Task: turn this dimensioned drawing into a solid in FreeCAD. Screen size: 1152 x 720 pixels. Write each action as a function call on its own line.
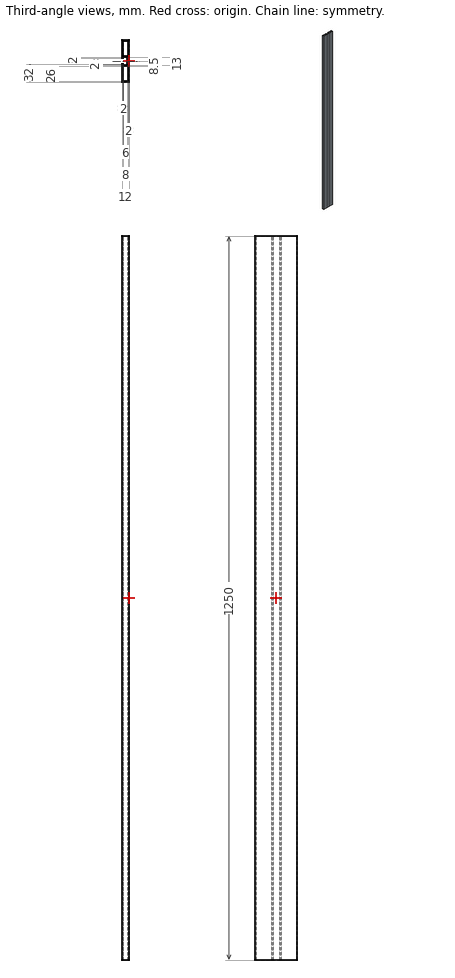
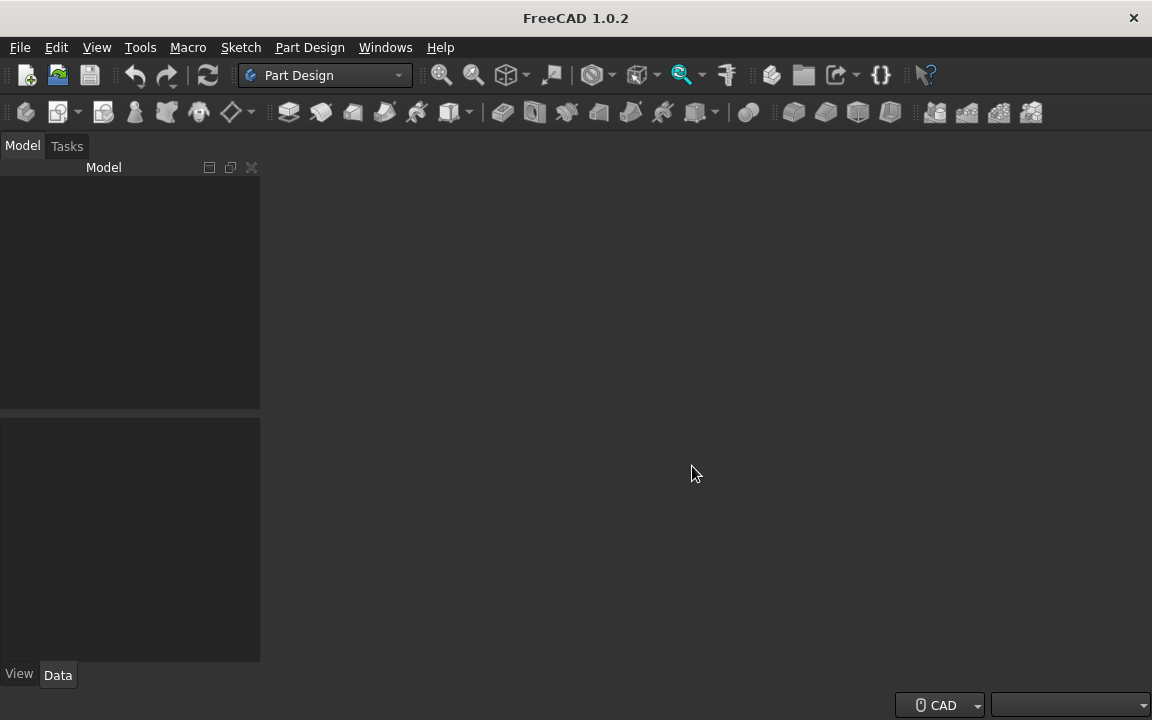
click(26, 76)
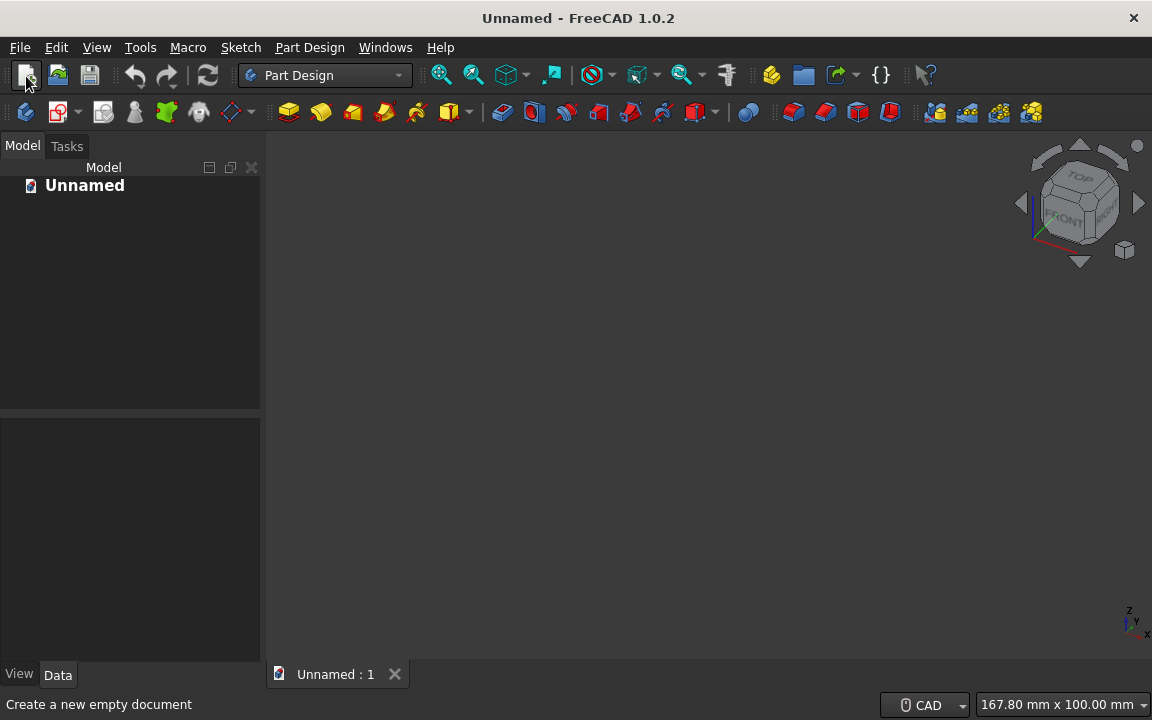
click(58, 112)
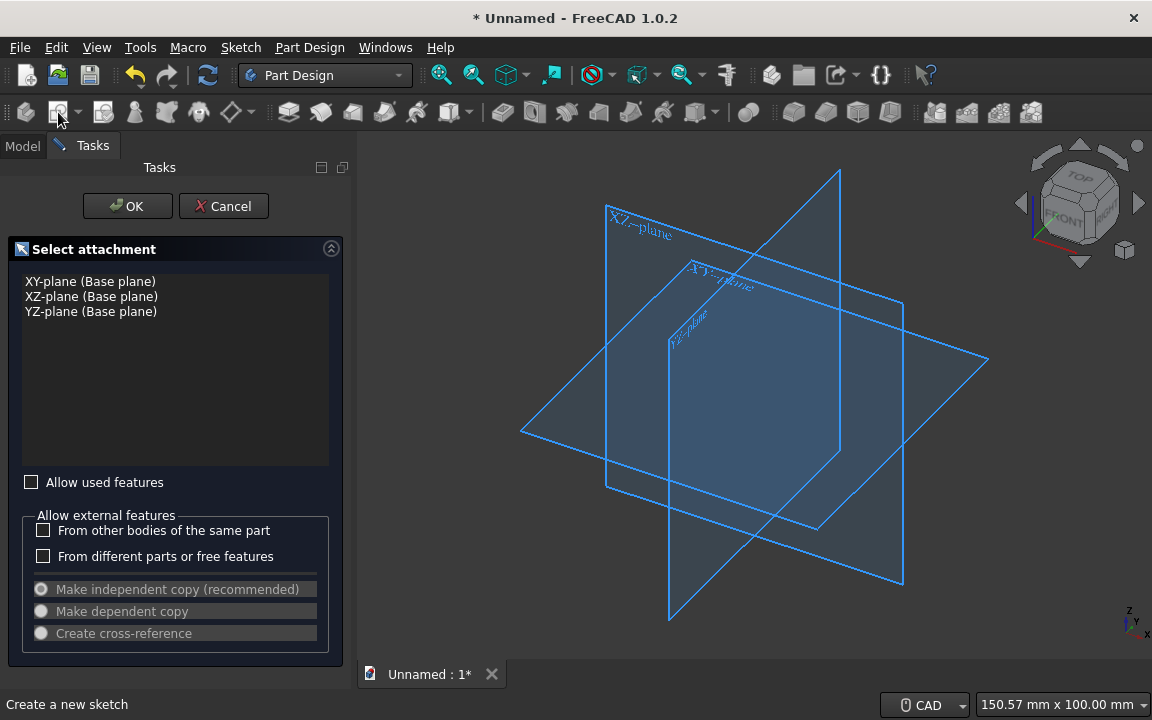
click(82, 282)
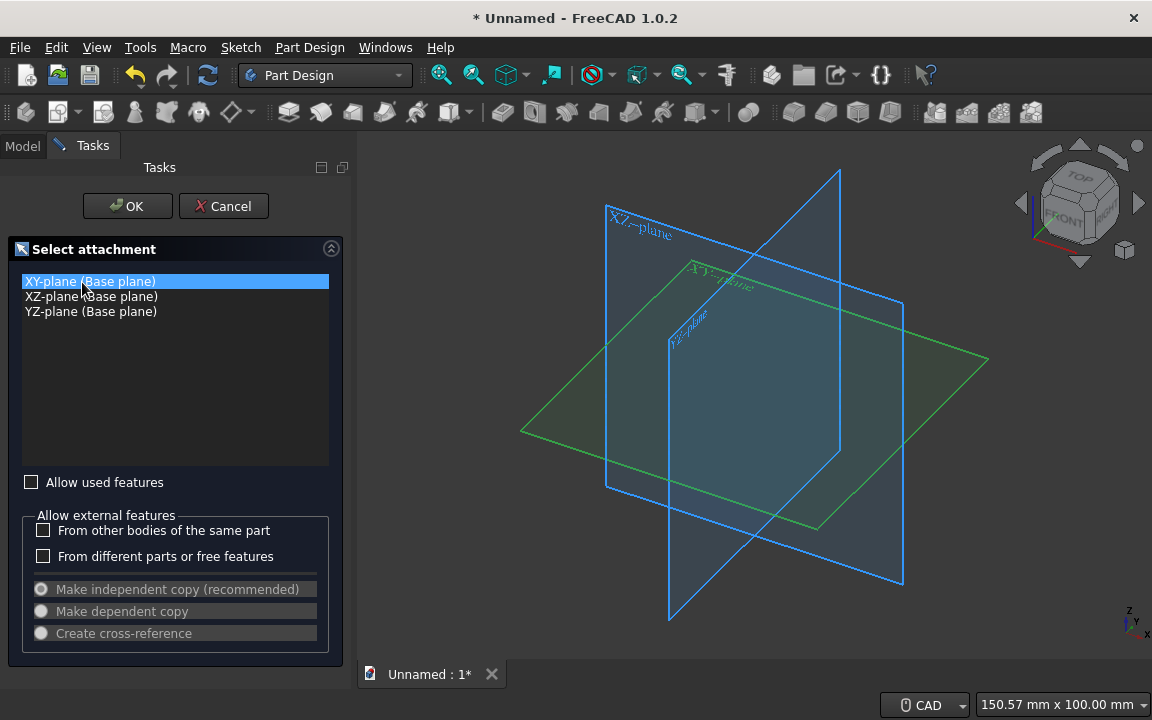
click(128, 206)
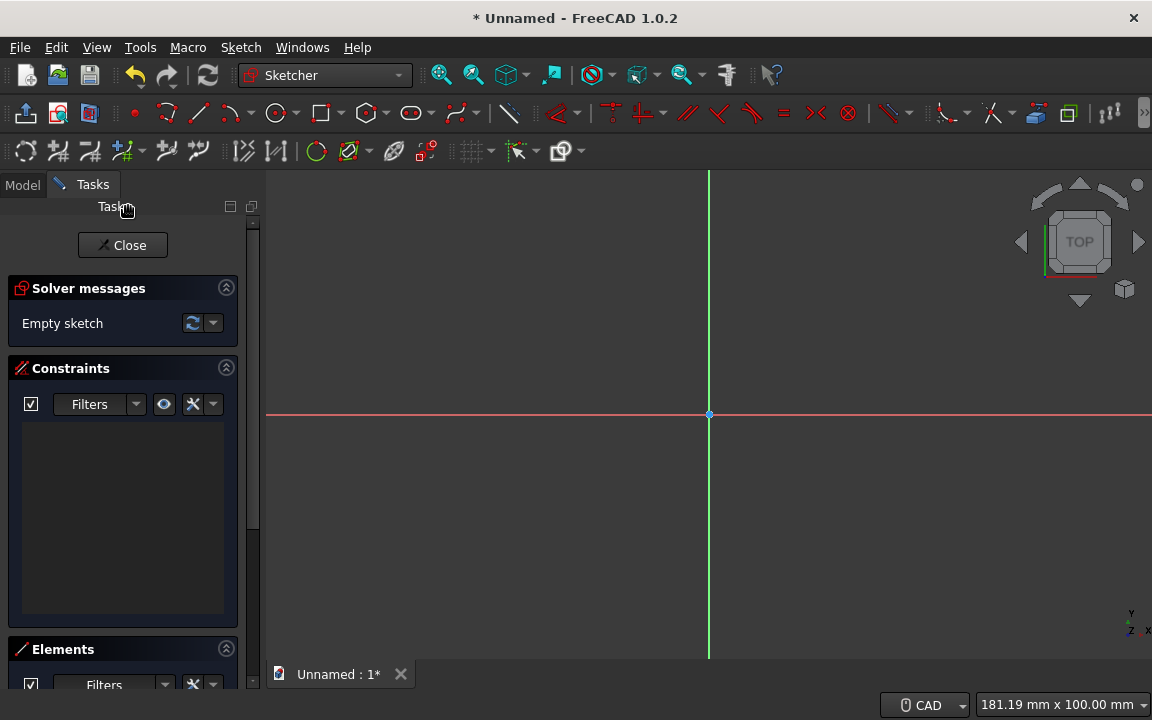
click(168, 114)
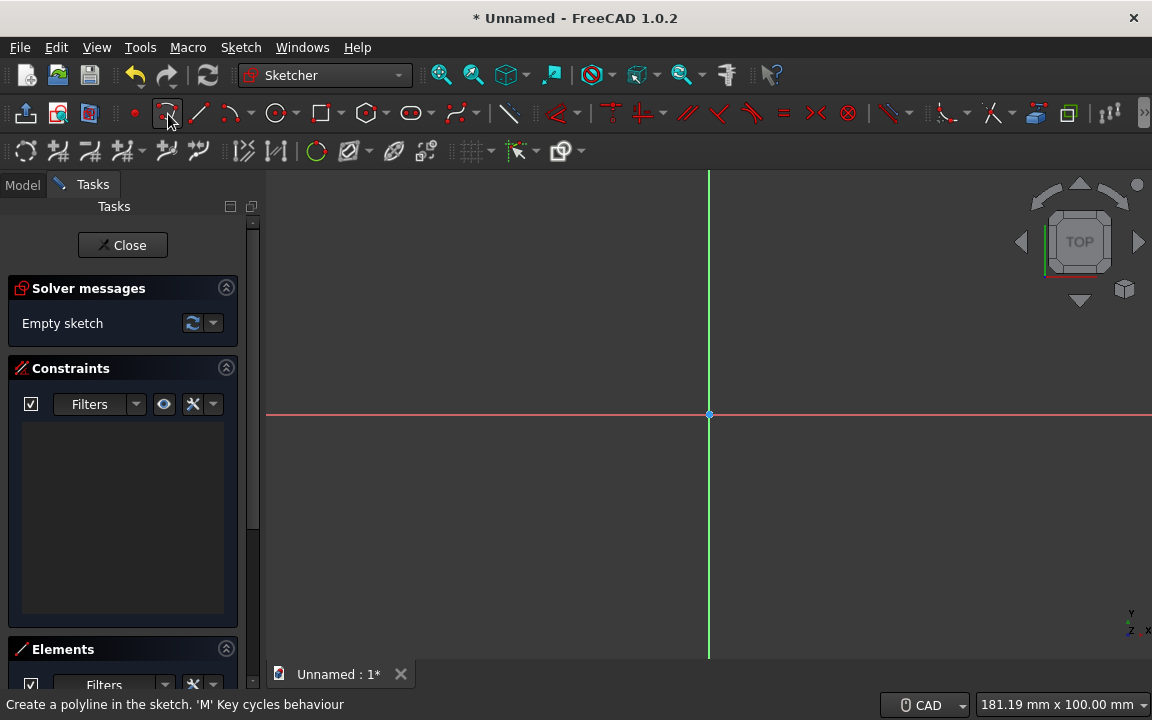
click(689, 383)
click(689, 446)
click(660, 446)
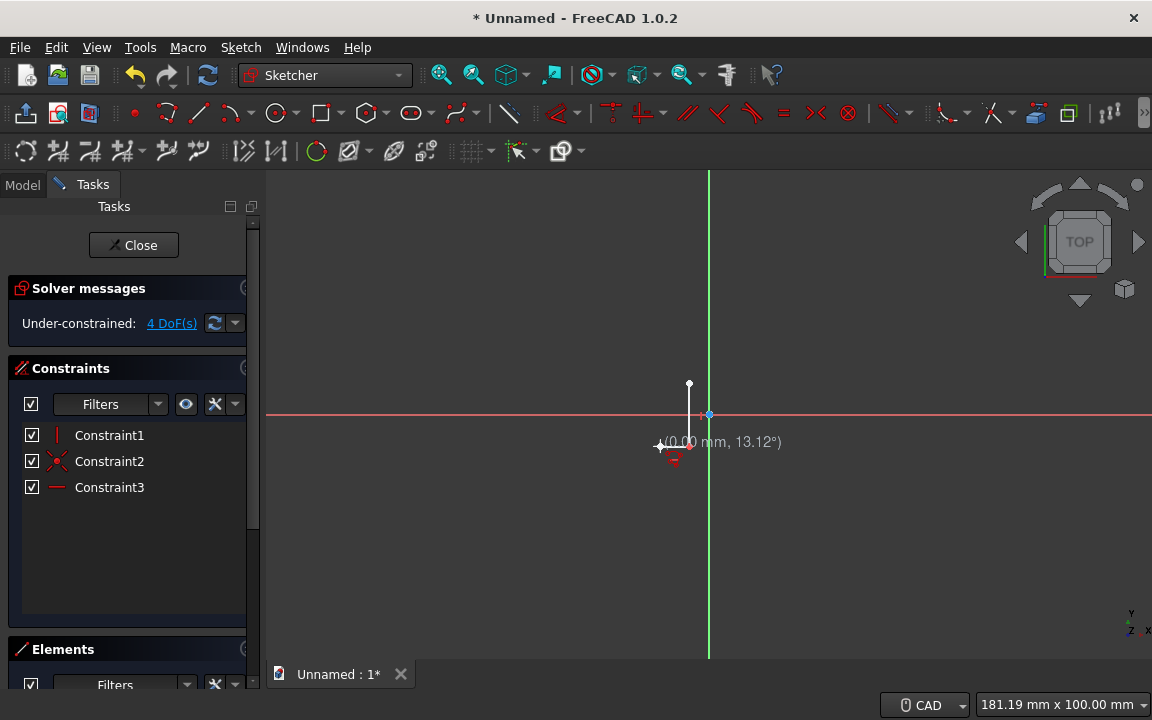
scroll(660, 437, up, 3)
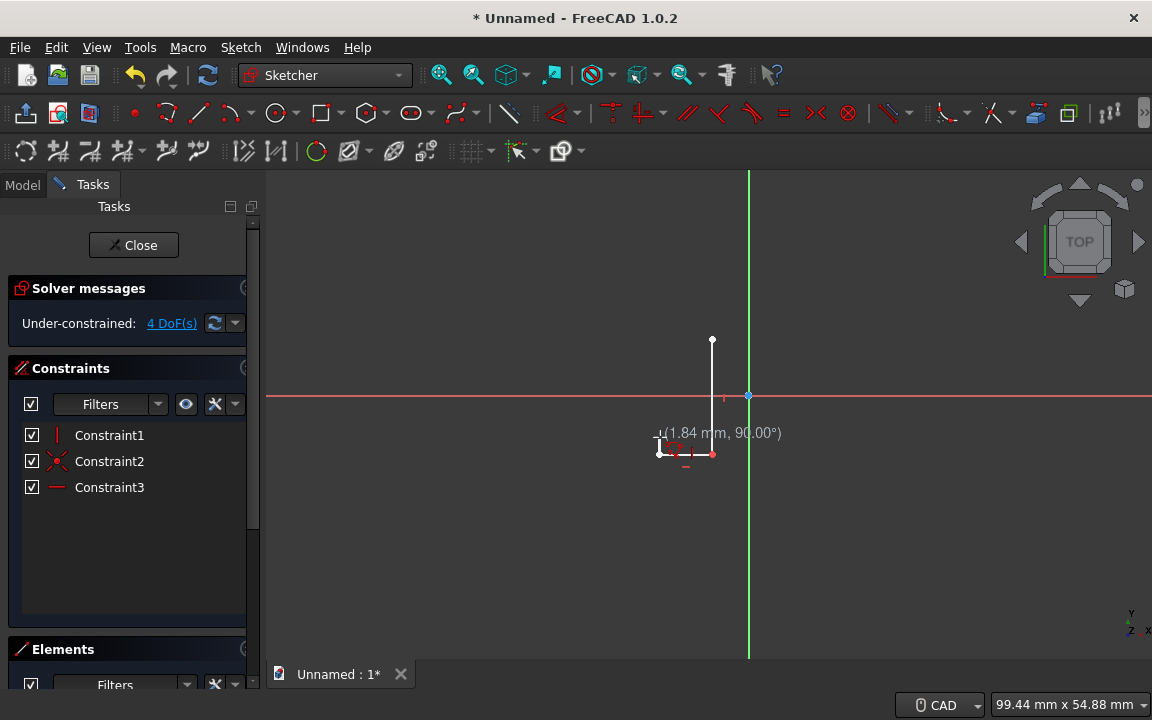
click(660, 436)
click(642, 436)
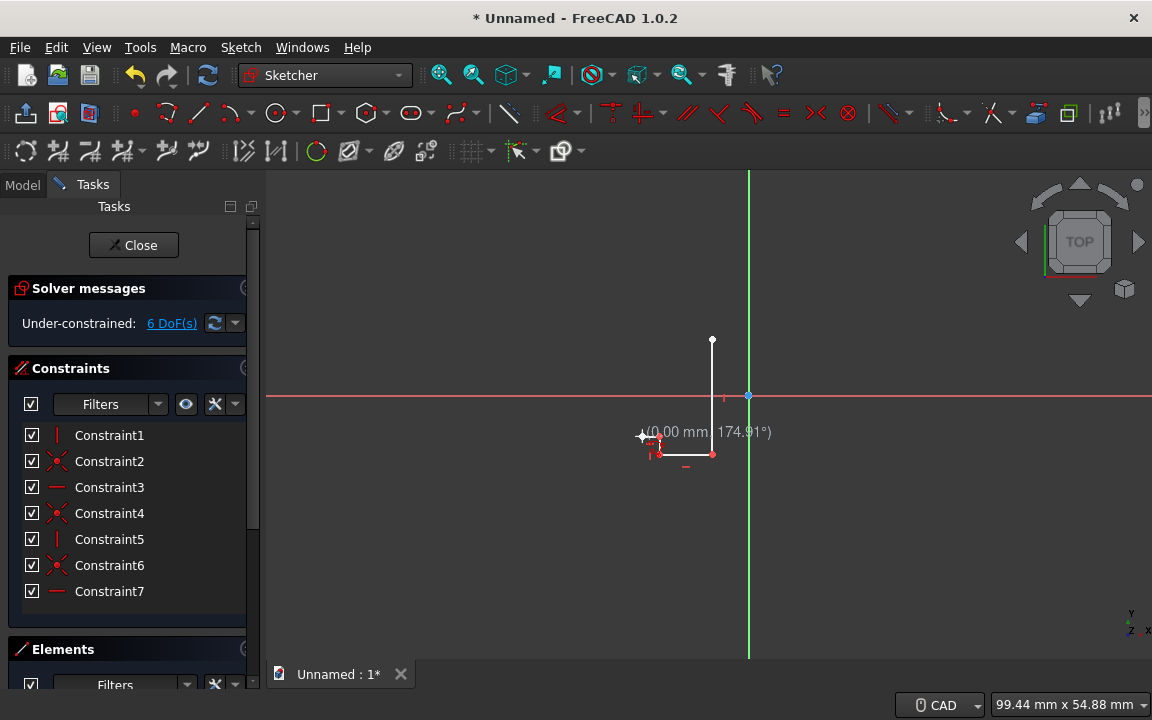
scroll(596, 430, down, 4)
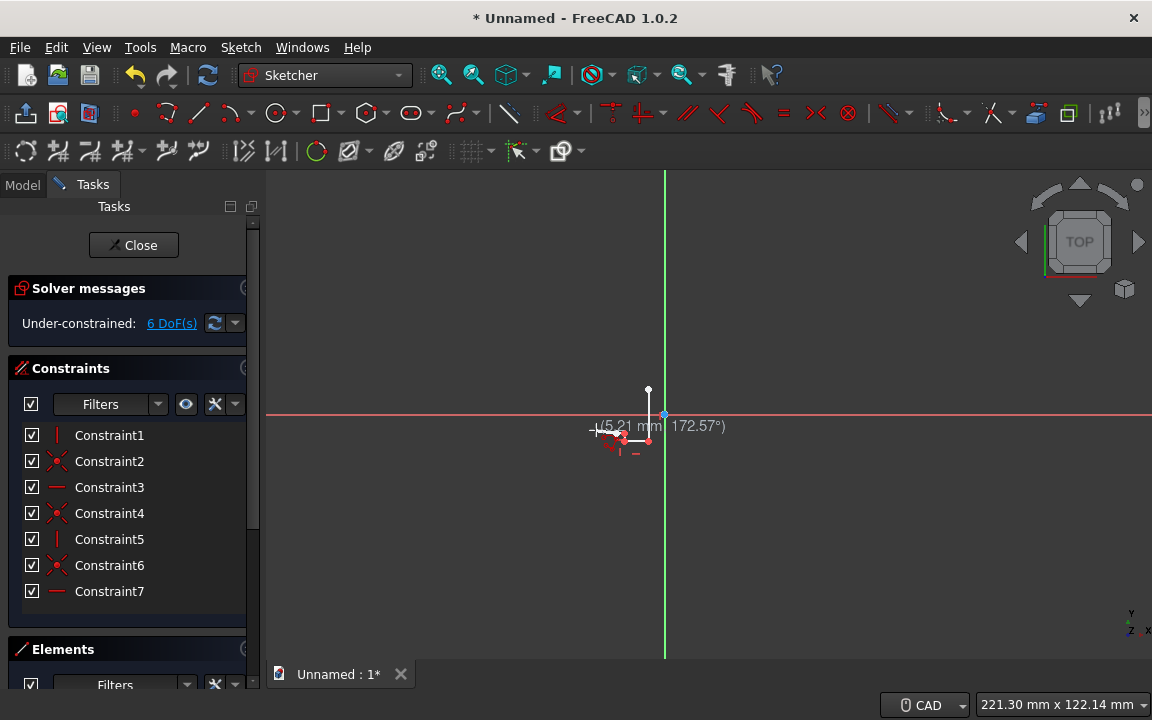
click(617, 561)
click(665, 561)
click(656, 269)
click(617, 269)
click(617, 397)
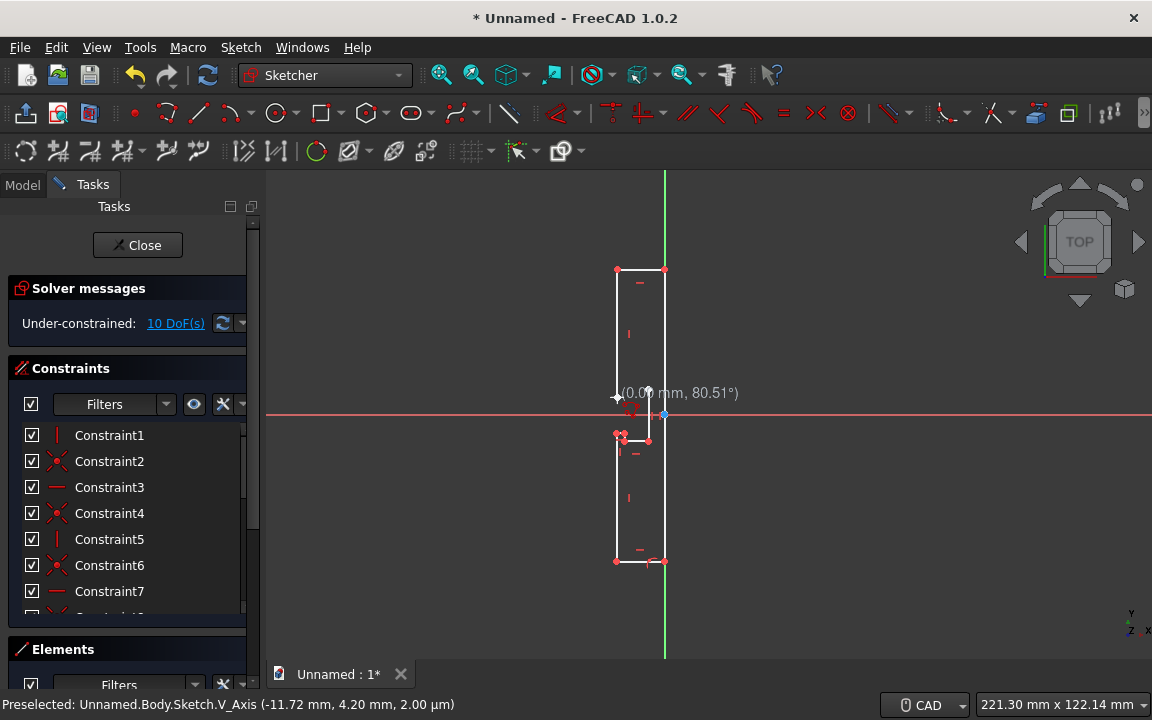
scroll(625, 397, up, 4)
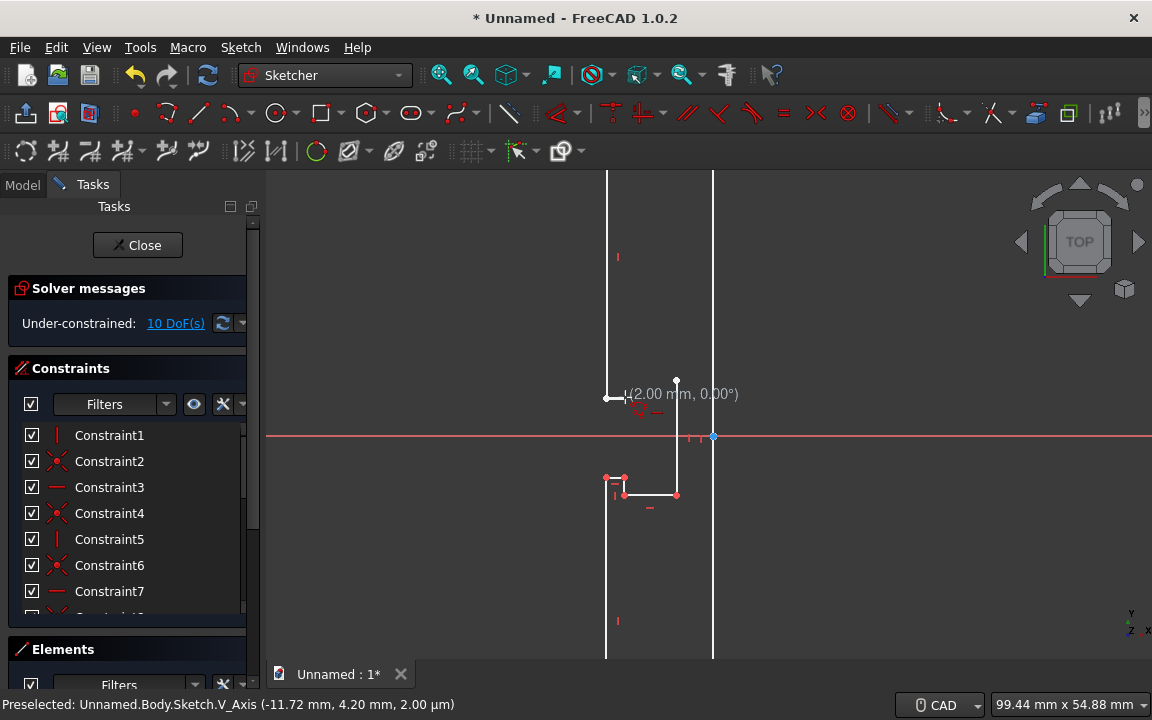
click(624, 396)
click(624, 378)
click(677, 381)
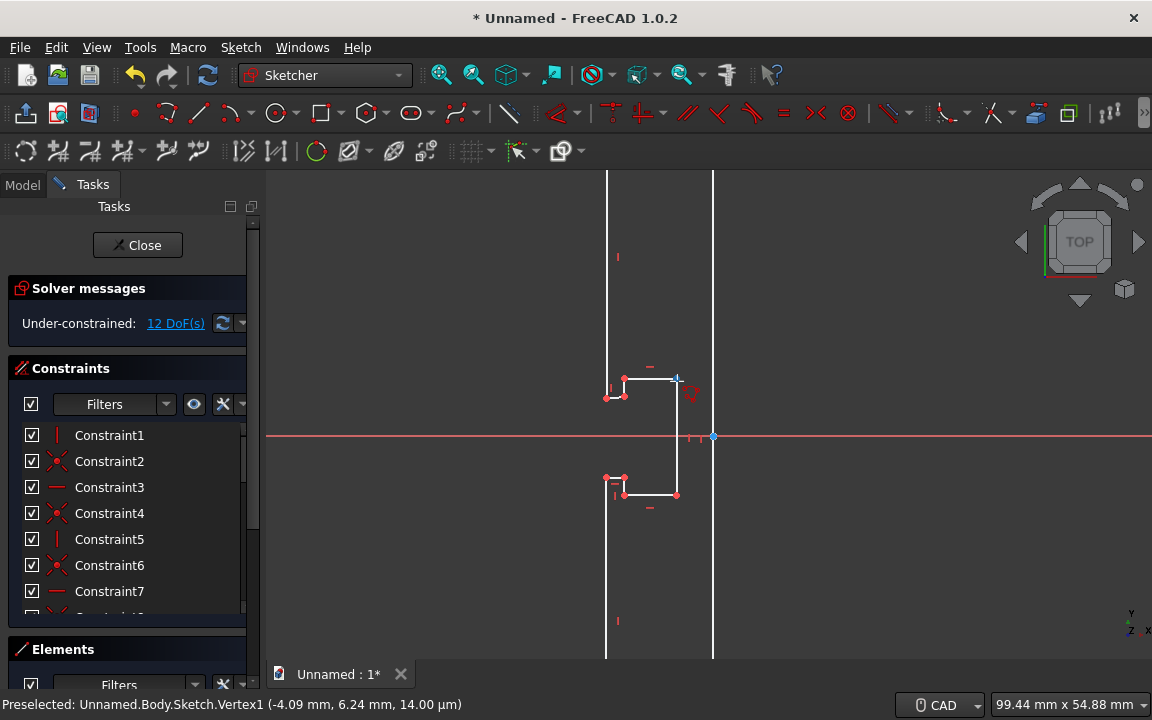
click(322, 114)